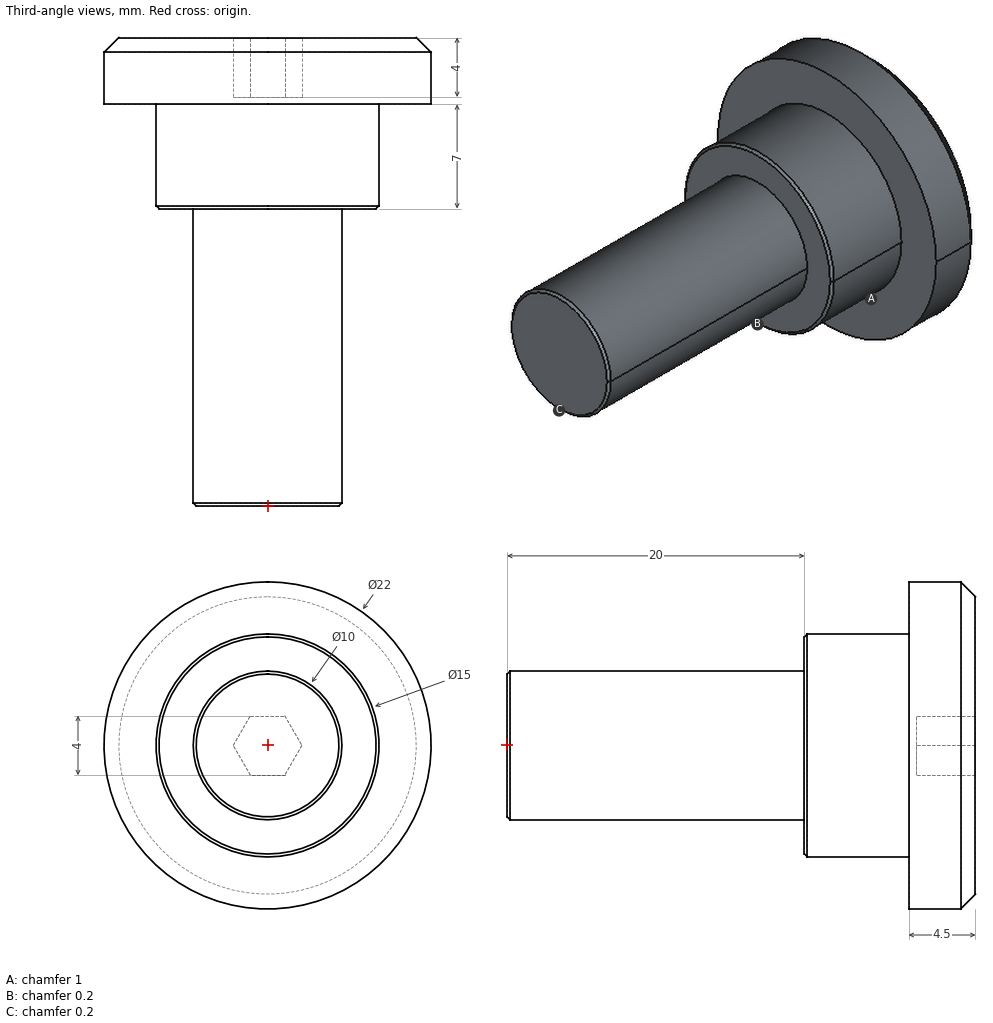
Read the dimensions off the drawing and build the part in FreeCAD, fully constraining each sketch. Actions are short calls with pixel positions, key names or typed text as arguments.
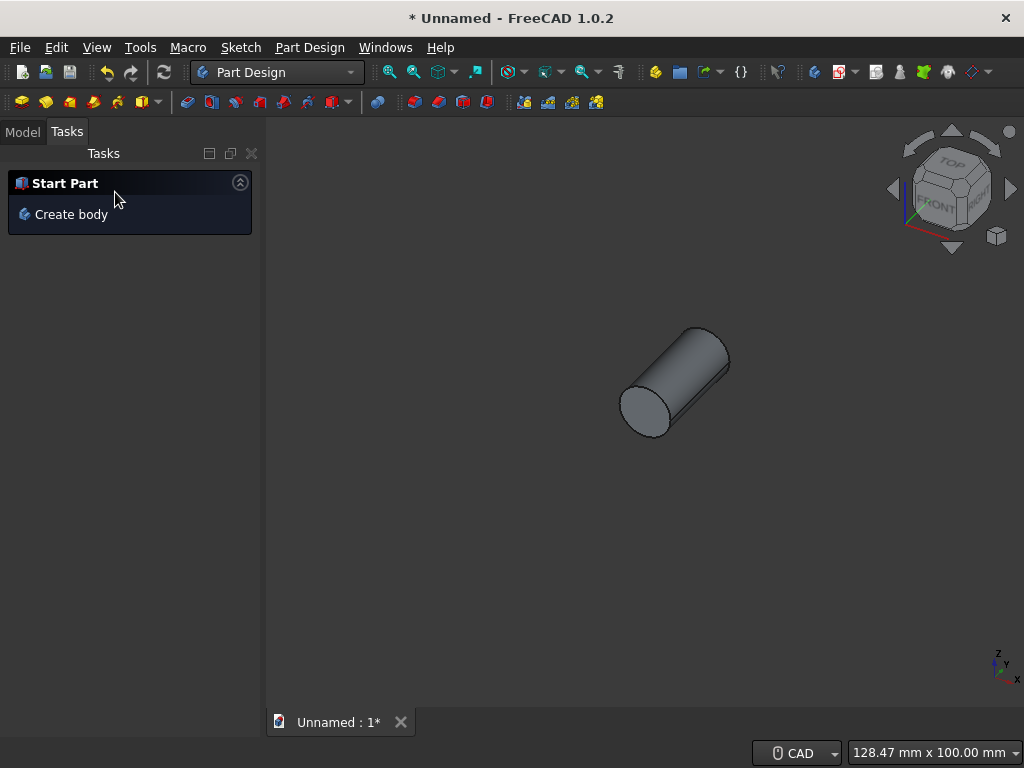
click(390, 72)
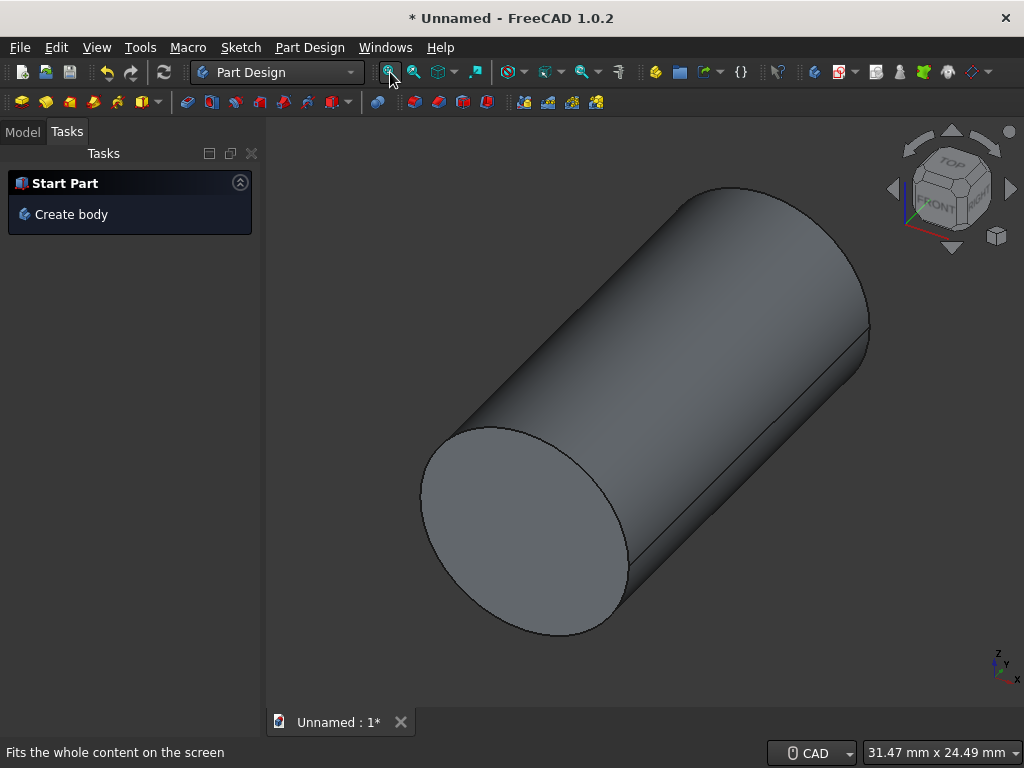
key(4)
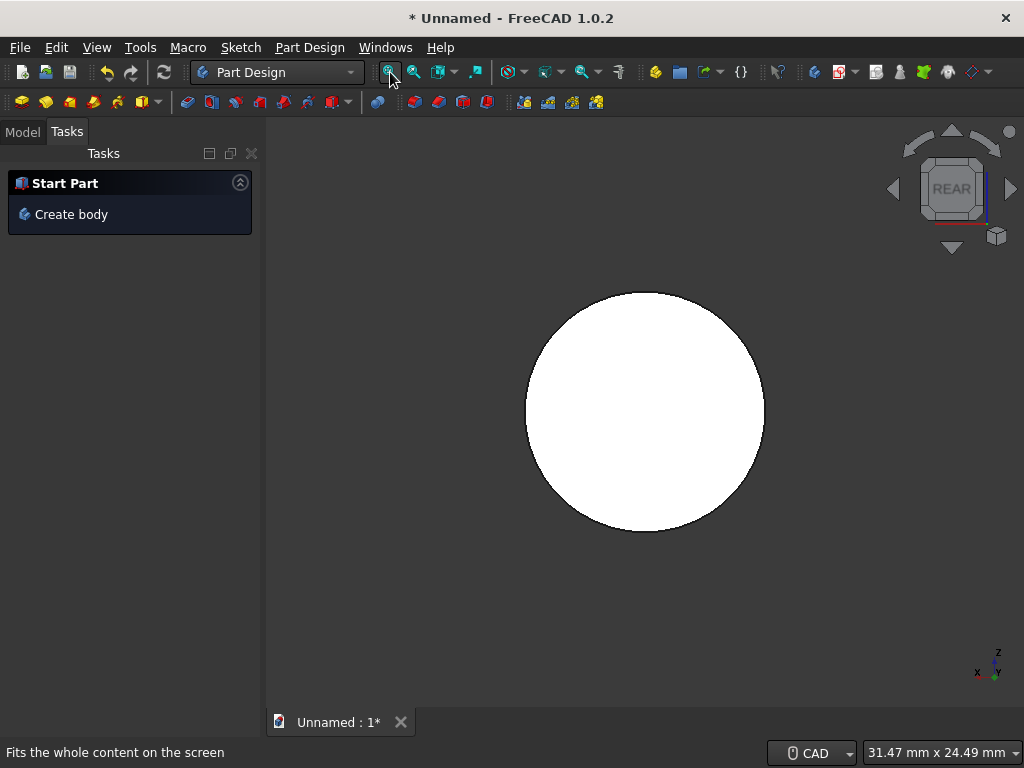
key(v)
key(f)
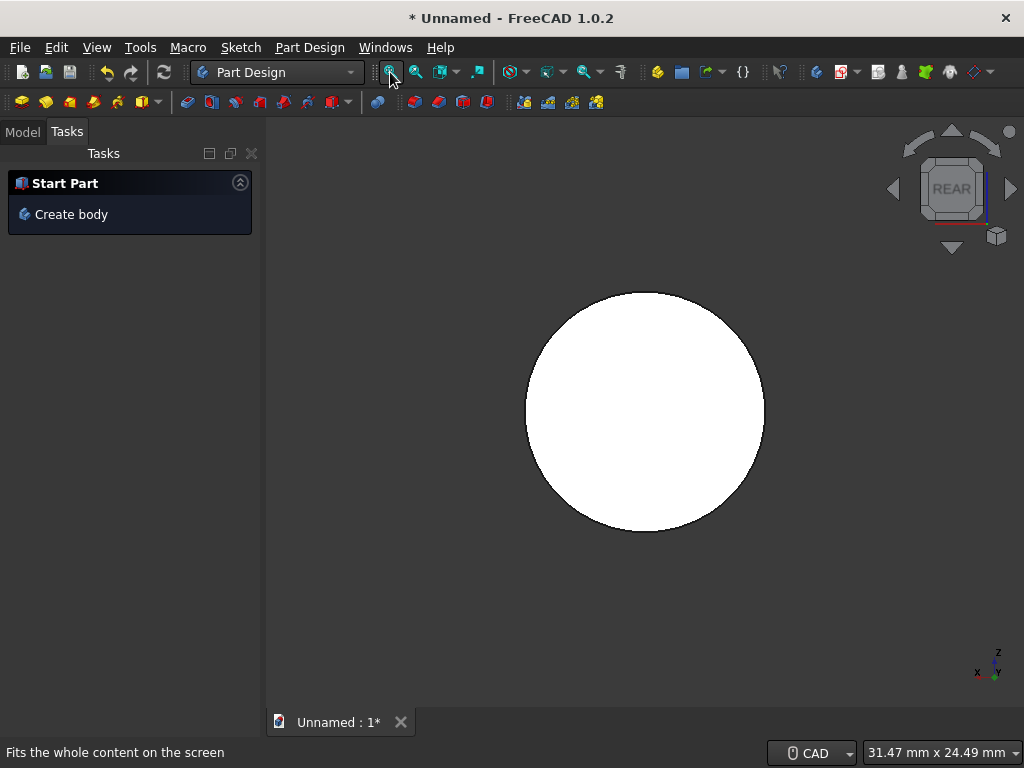
click(645, 411)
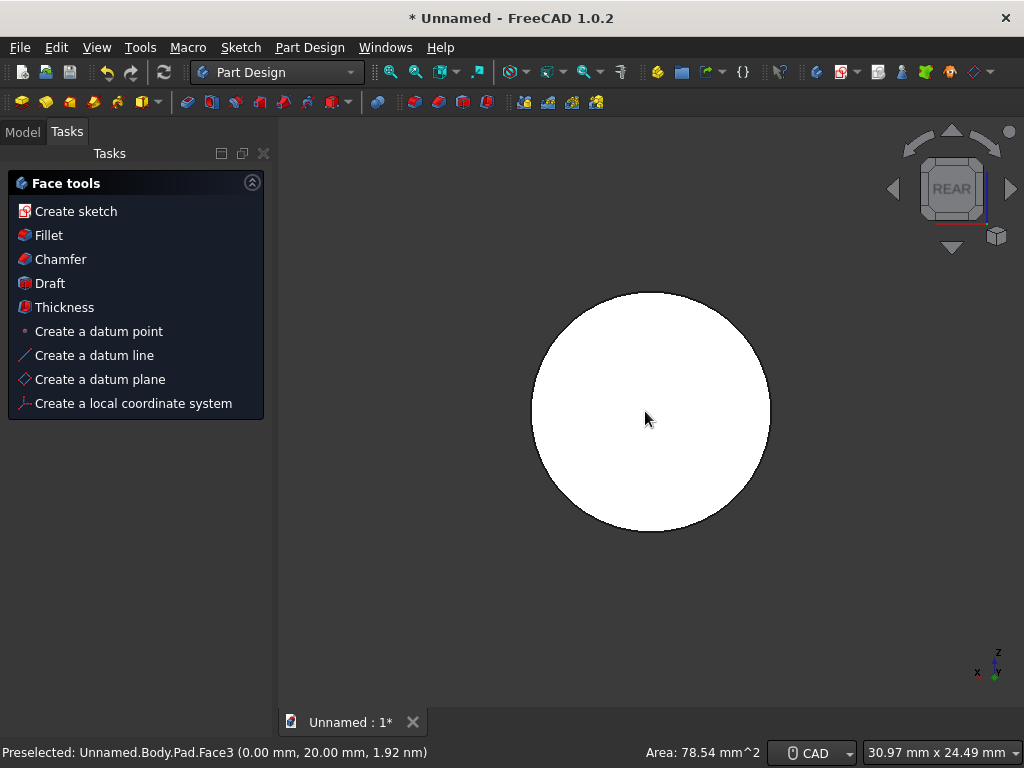
click(842, 72)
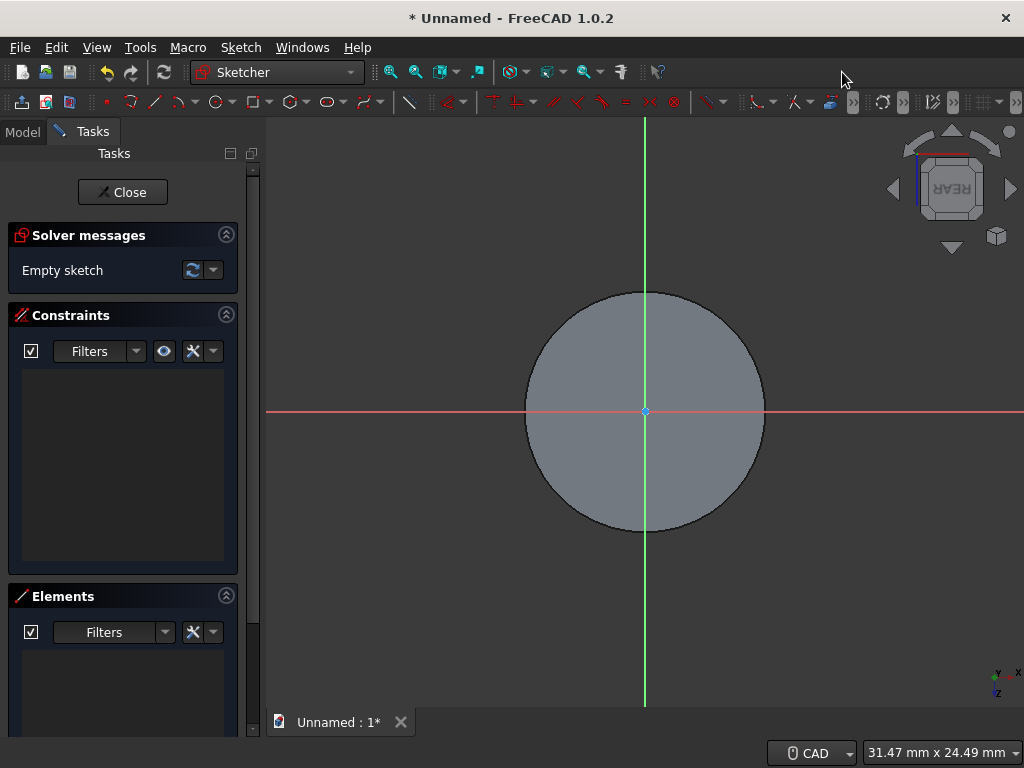
click(216, 102)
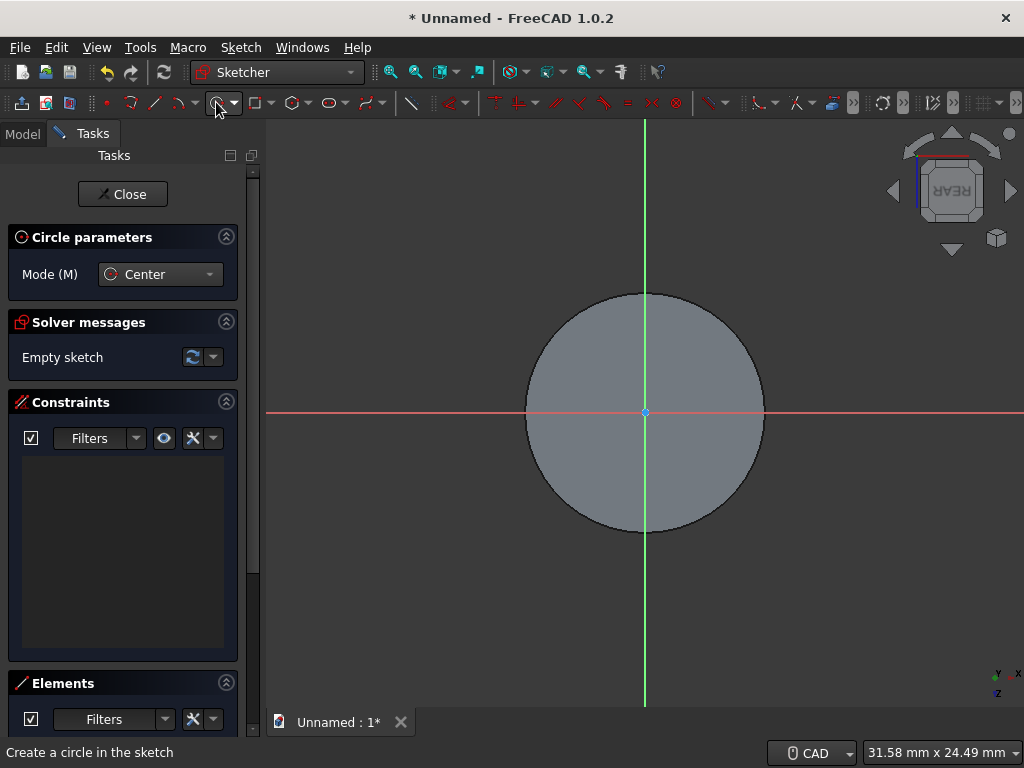
click(645, 413)
move(772, 286)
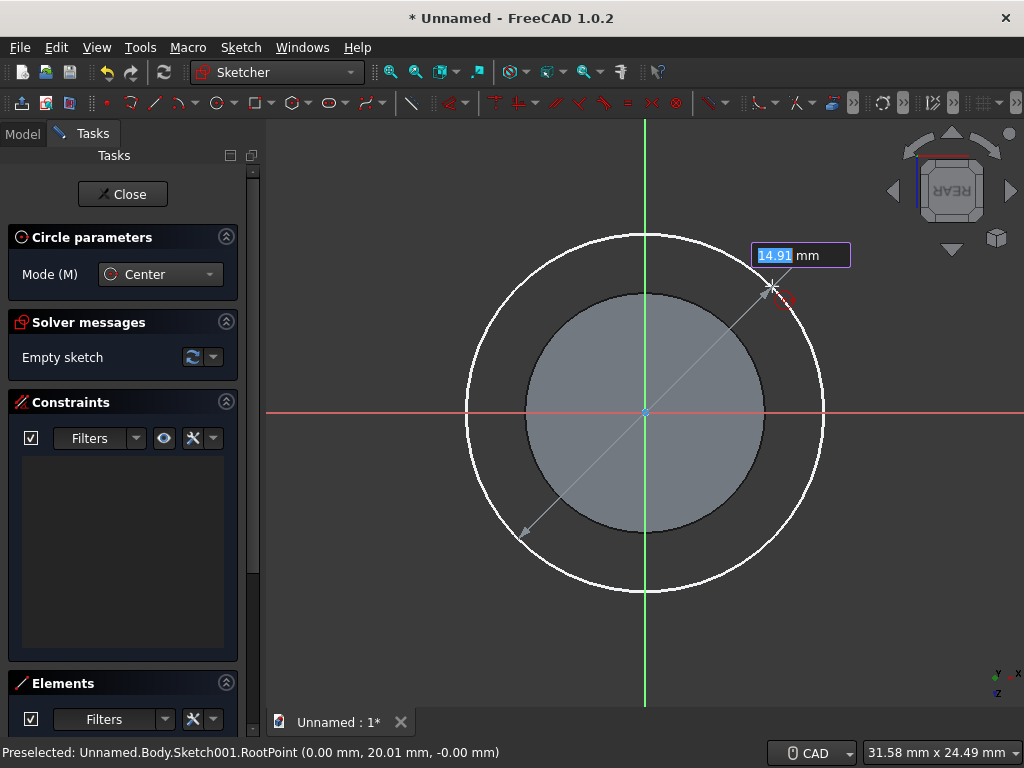
text(15)
key(Return)
key(Escape)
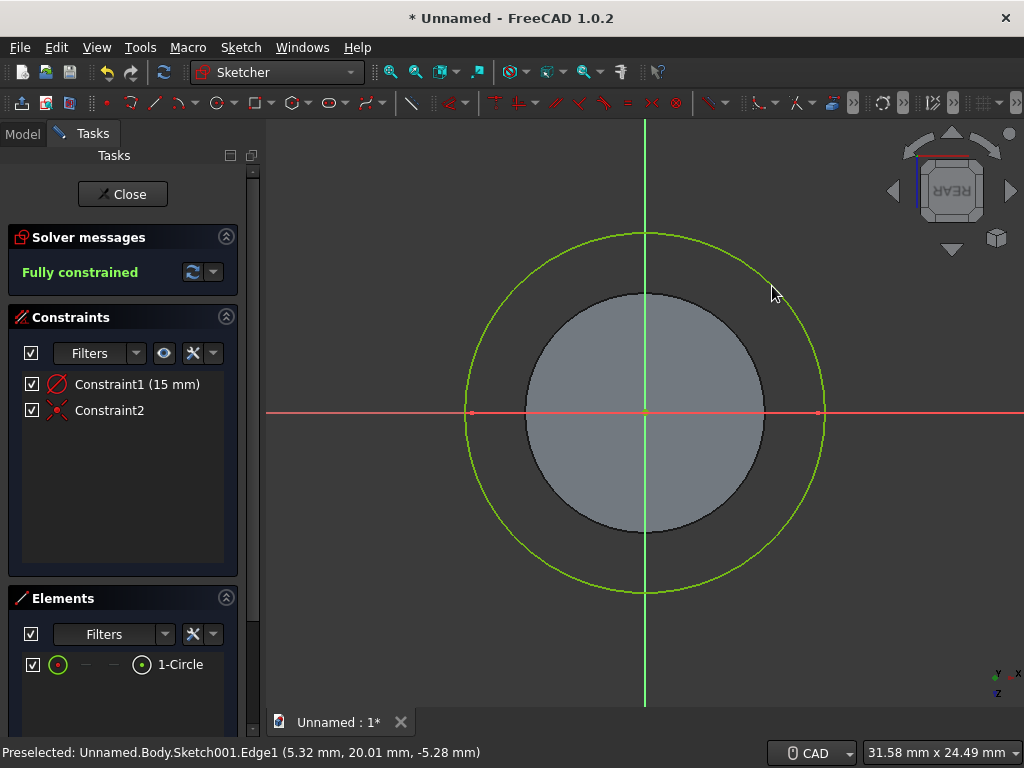
click(123, 194)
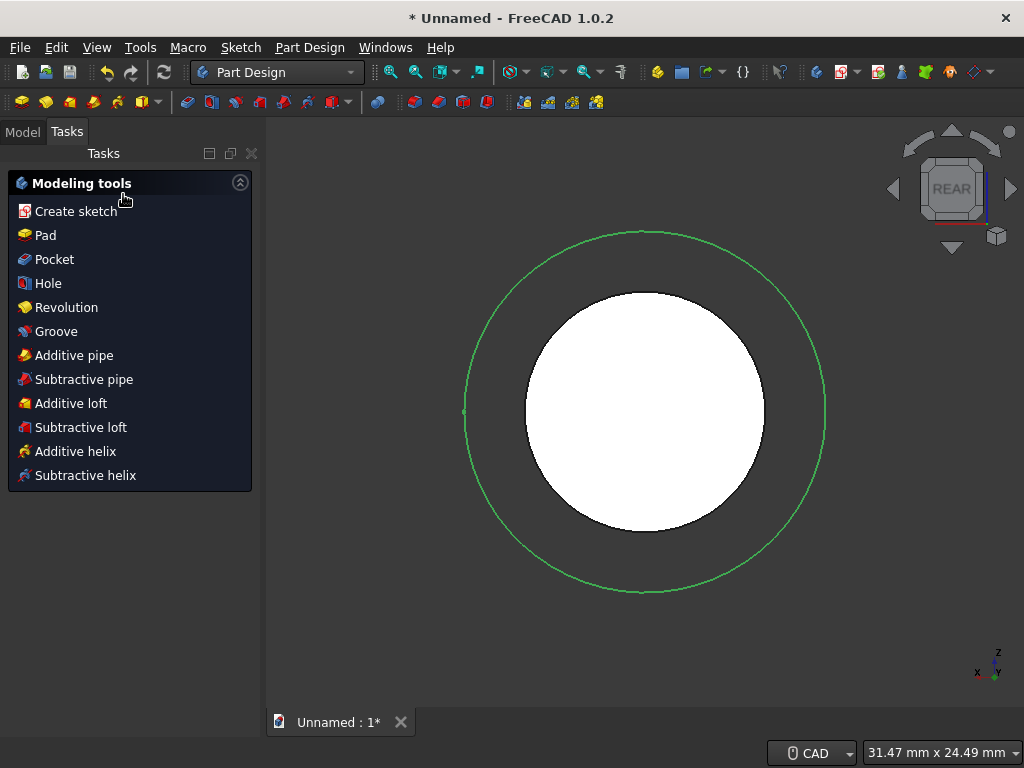
click(22, 102)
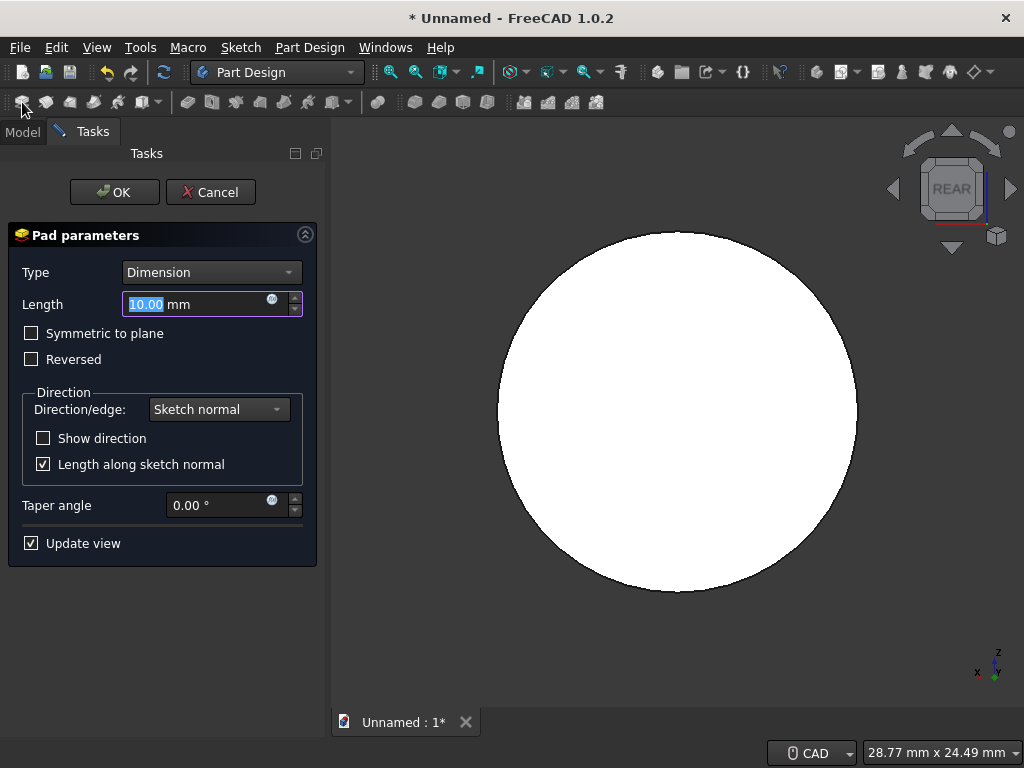
text(7)
key(Tab)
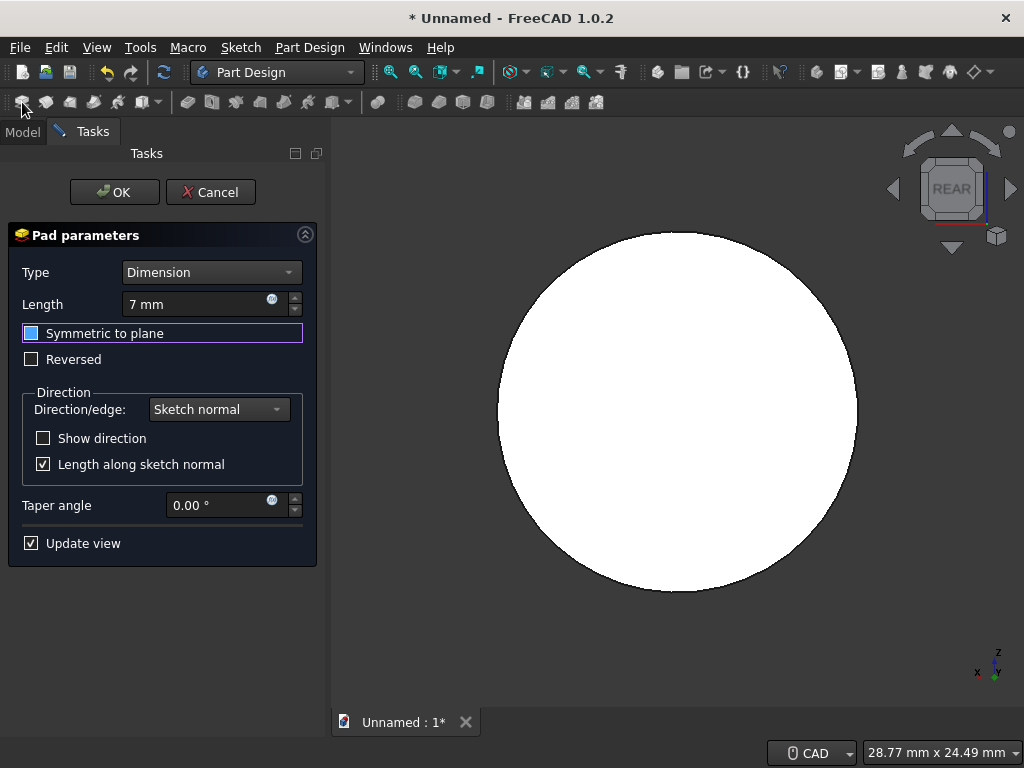
click(115, 192)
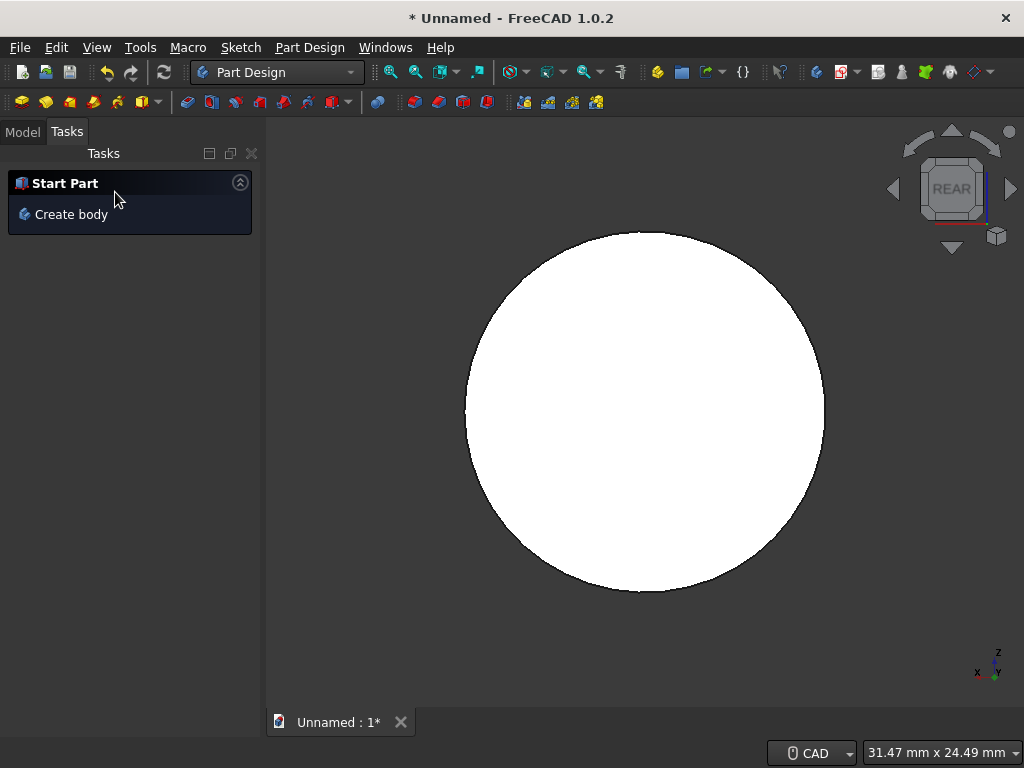
click(645, 411)